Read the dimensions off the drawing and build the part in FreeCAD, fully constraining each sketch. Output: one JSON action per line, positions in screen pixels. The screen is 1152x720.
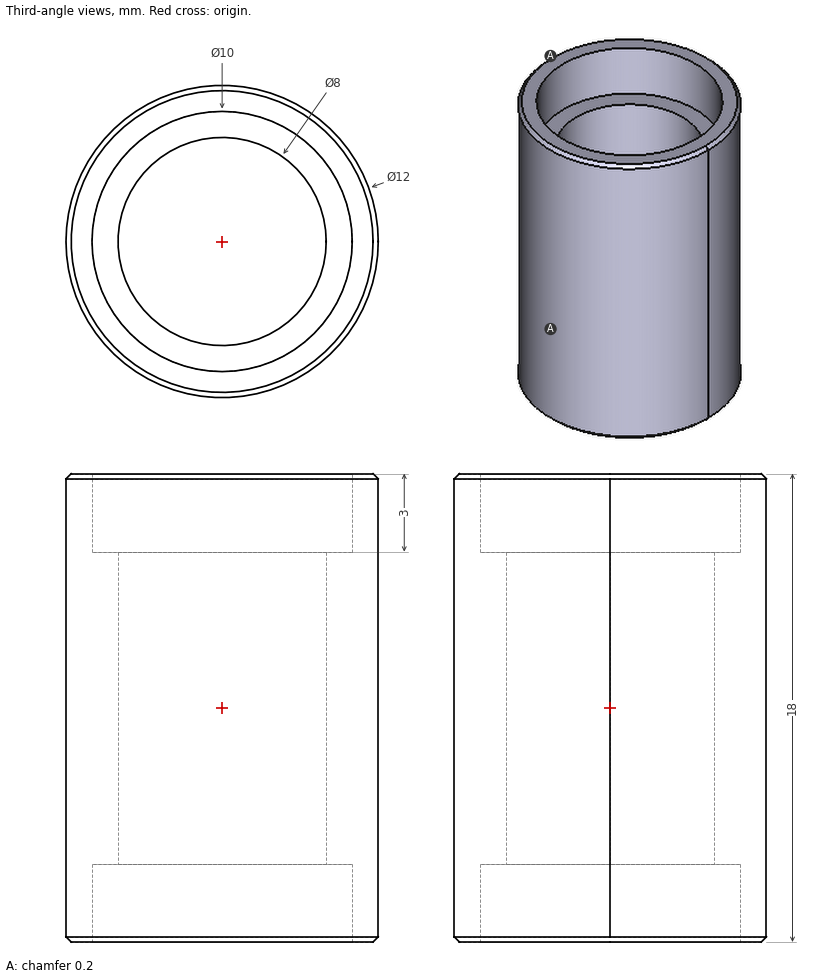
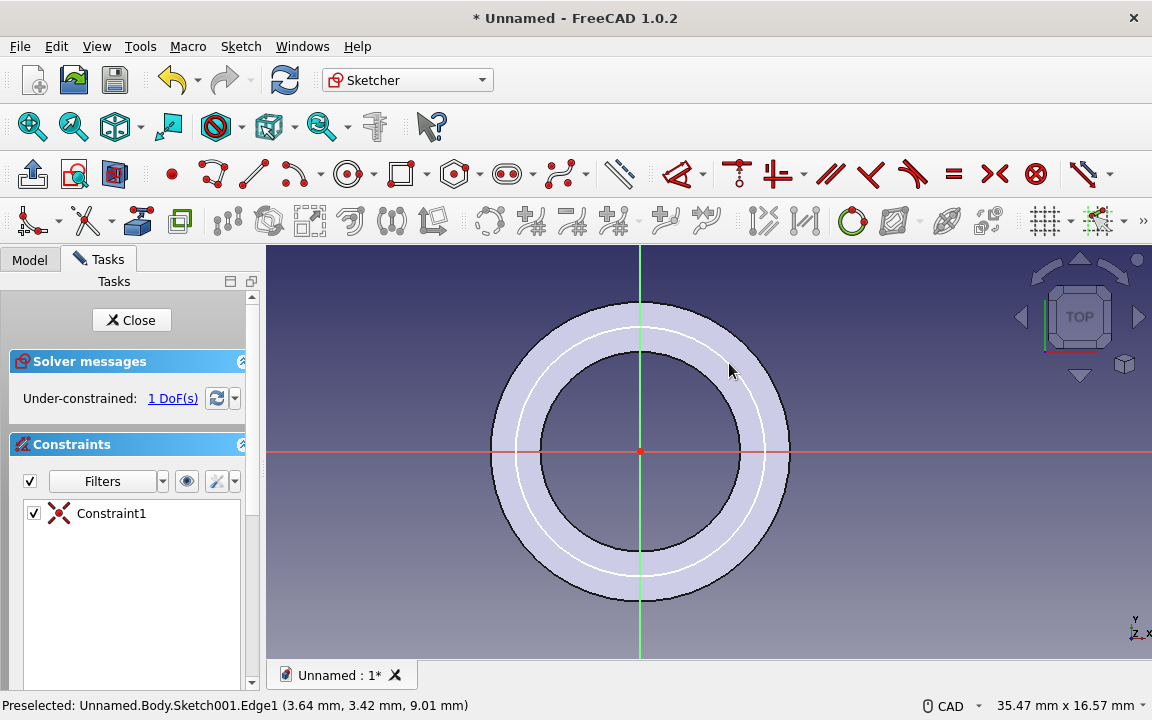
{"action": "left_click", "coordinate": [676, 174]}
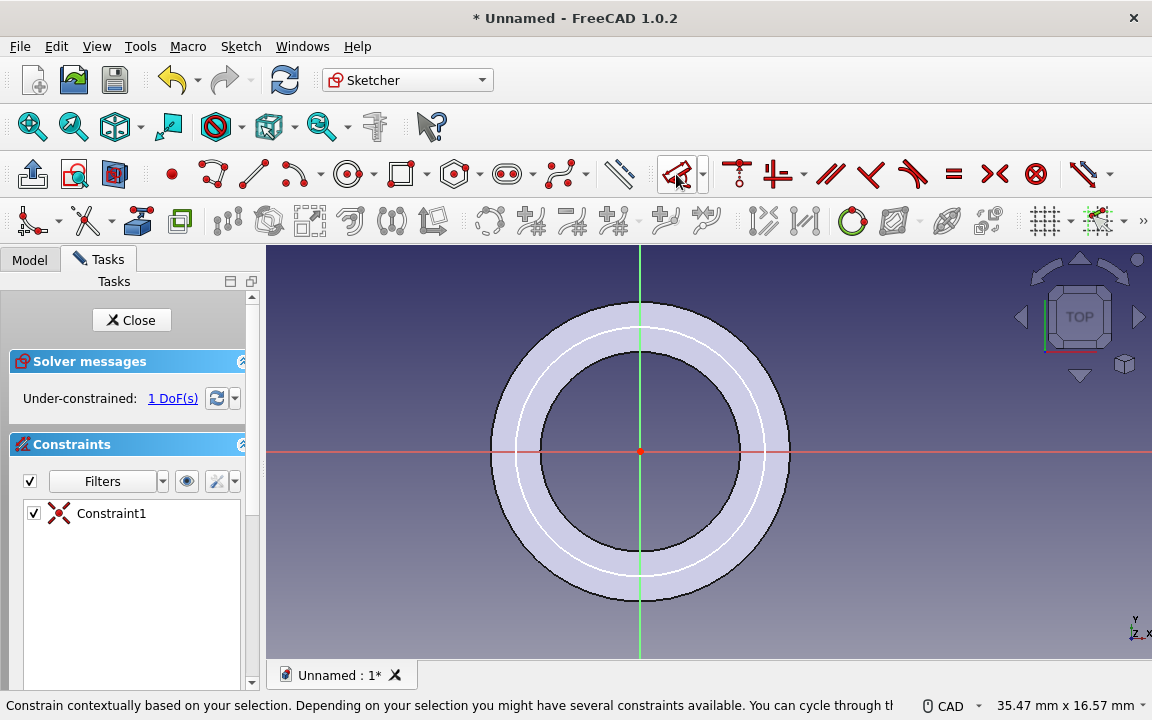
{"action": "left_click", "coordinate": [728, 363]}
{"action": "left_click", "coordinate": [750, 340]}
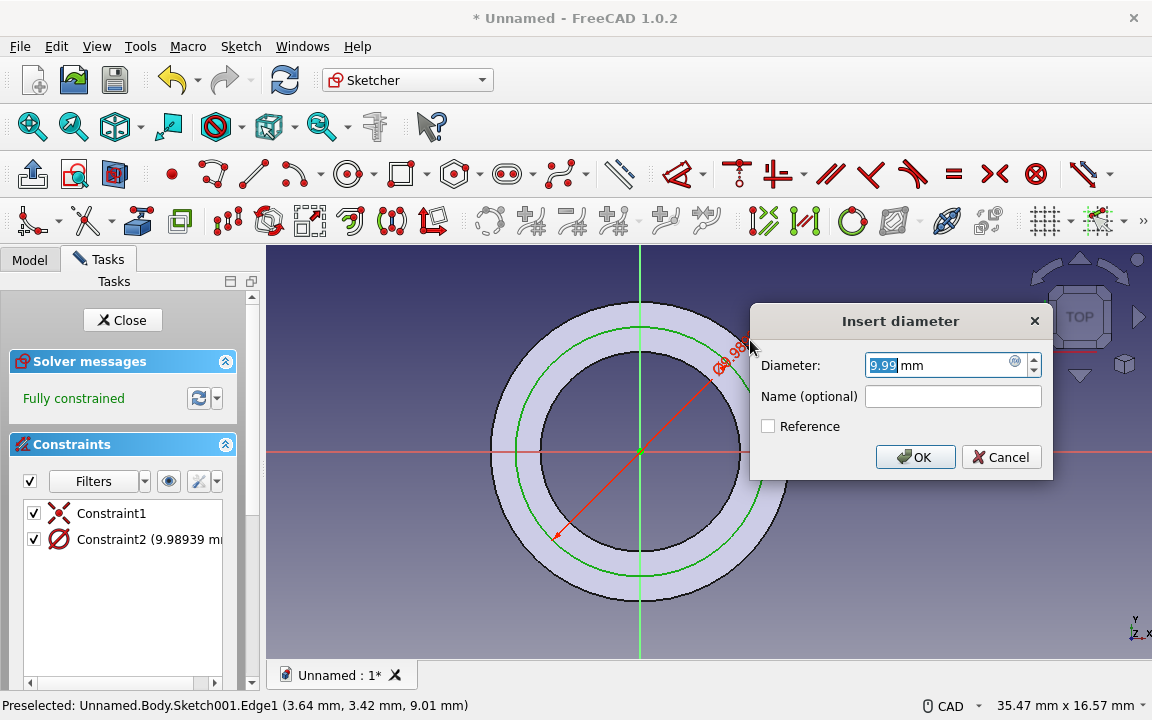
{"action": "type", "text": "10"}
{"action": "key", "text": "Return"}
{"action": "key", "text": "Escape"}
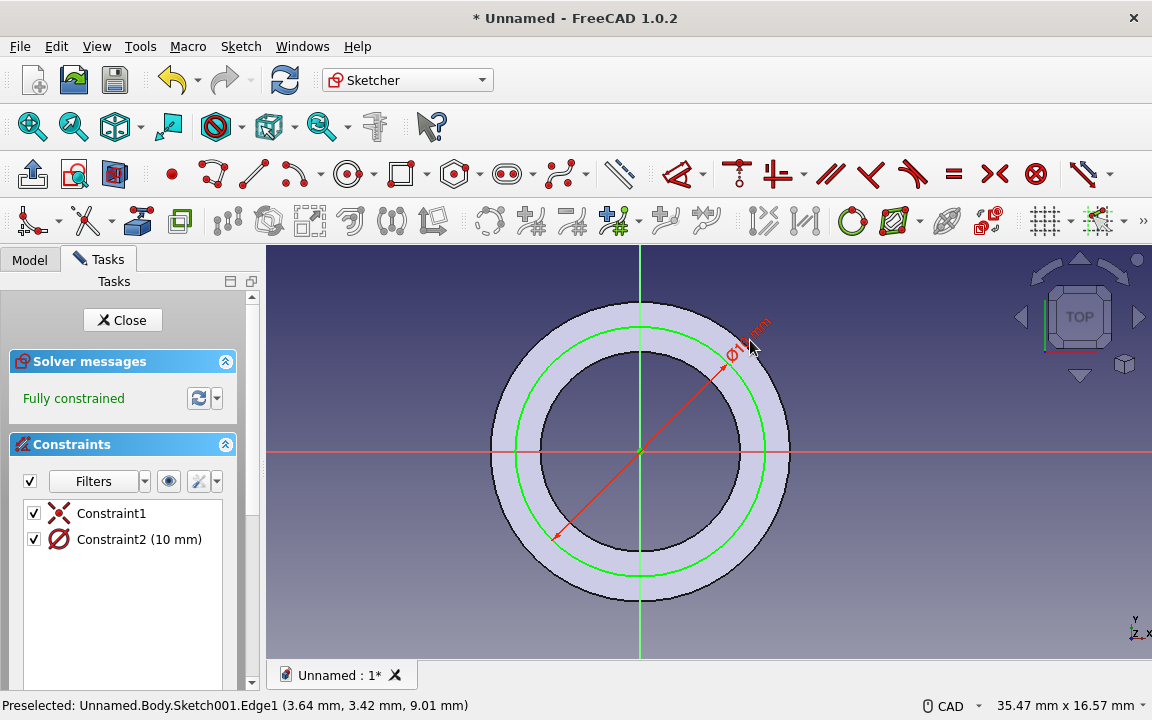
{"action": "left_click", "coordinate": [123, 320]}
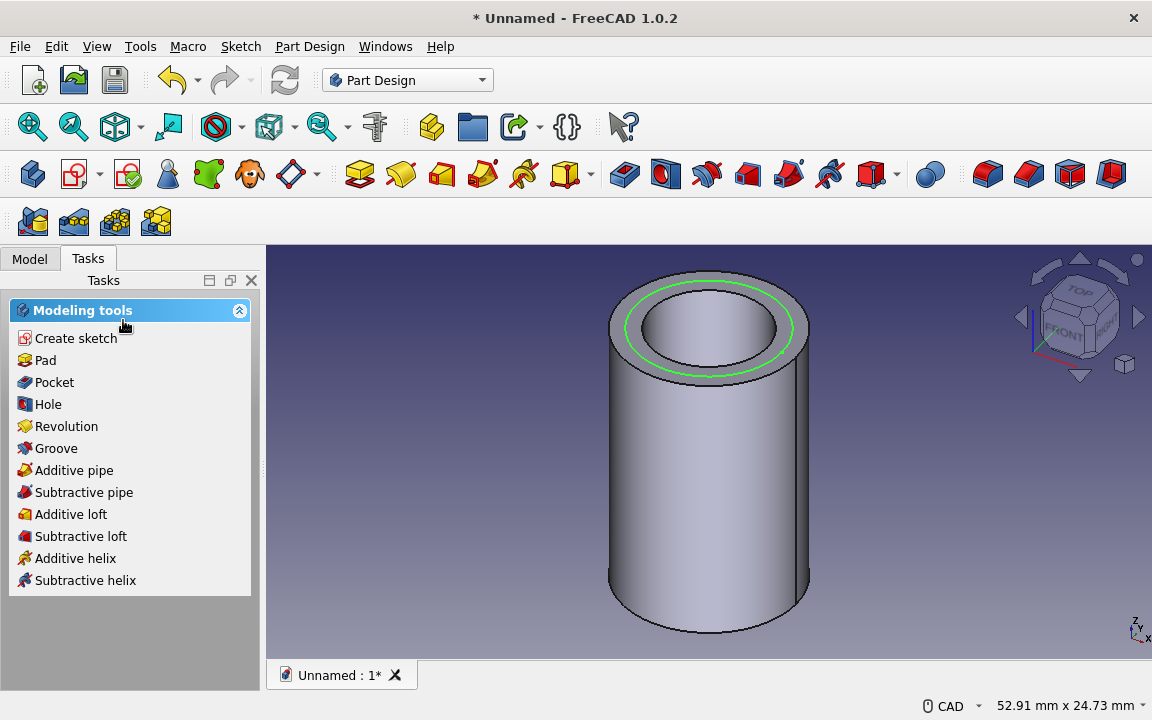
{"action": "left_click", "coordinate": [625, 174]}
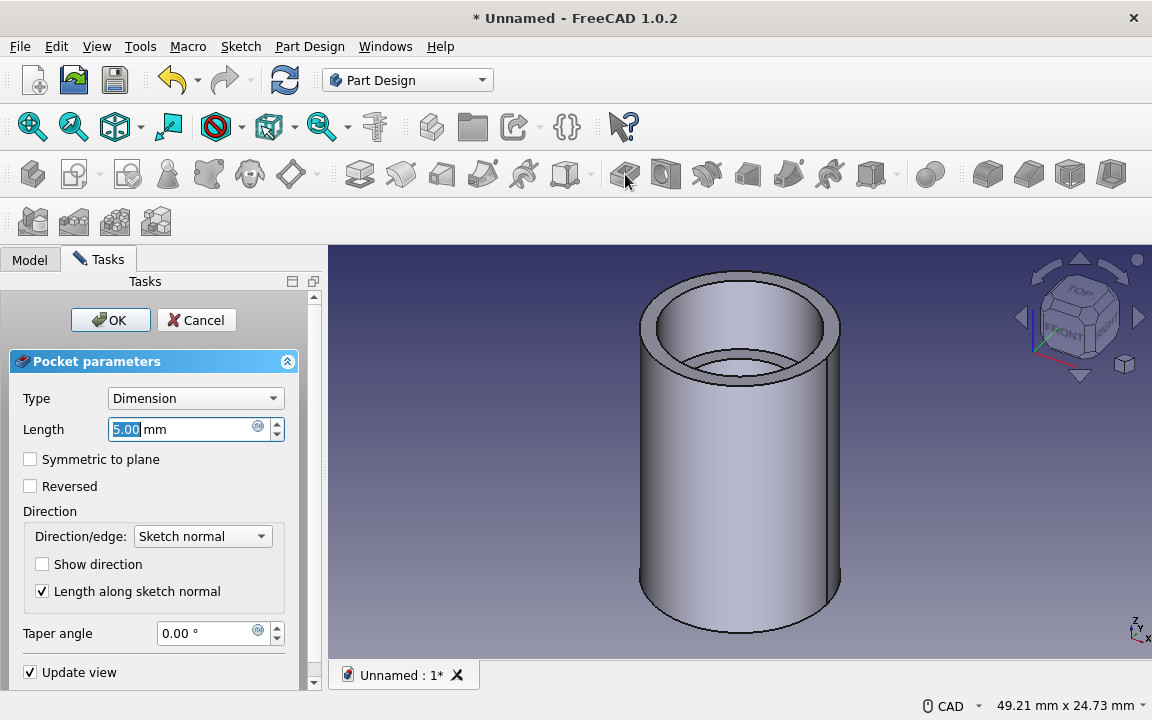
{"action": "type", "text": "3"}
{"action": "key", "text": "Tab"}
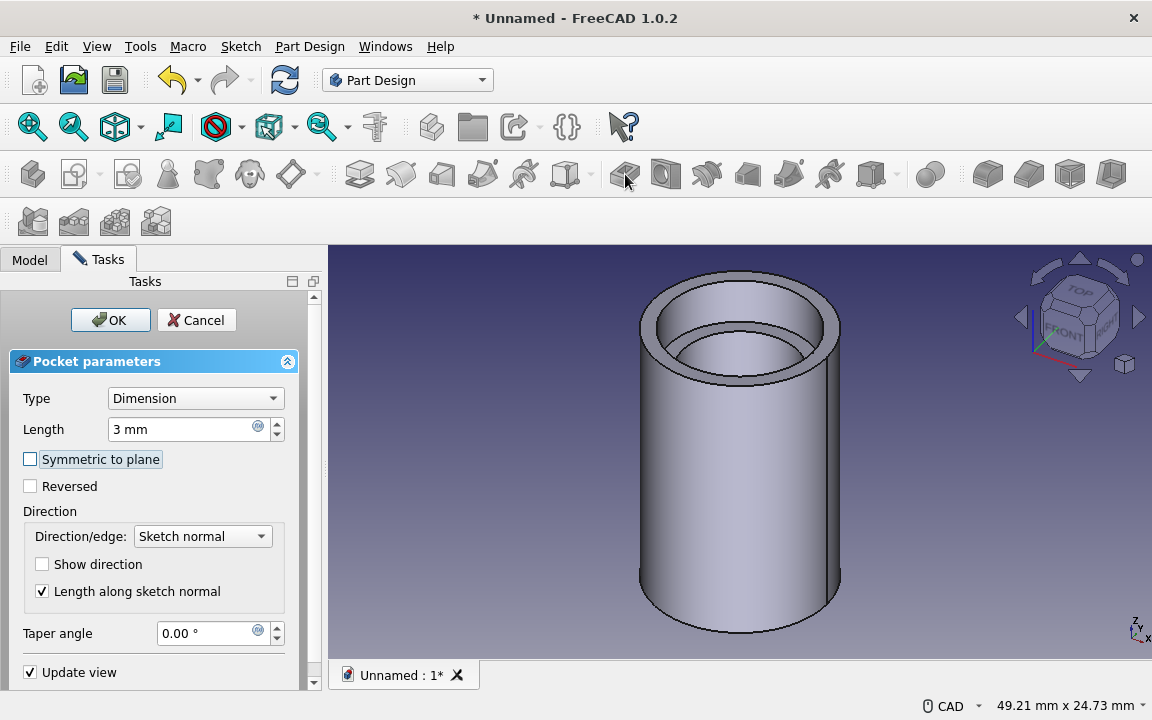
{"action": "left_click", "coordinate": [111, 320]}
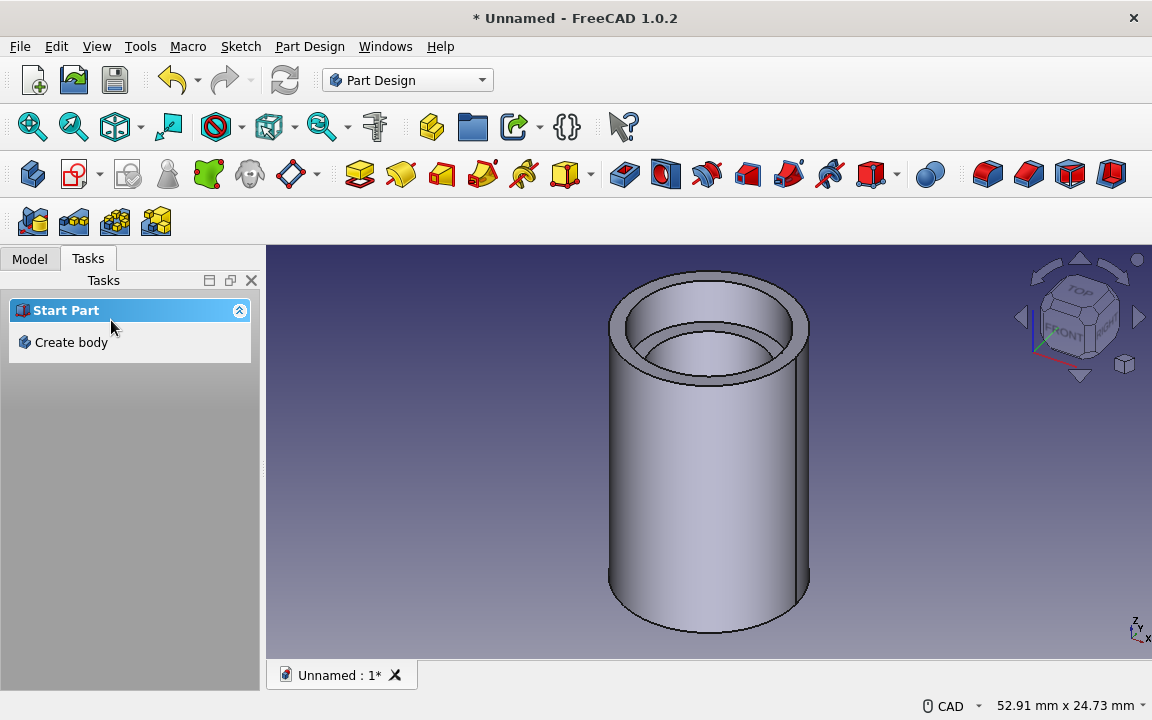
{"action": "left_click", "coordinate": [30, 258]}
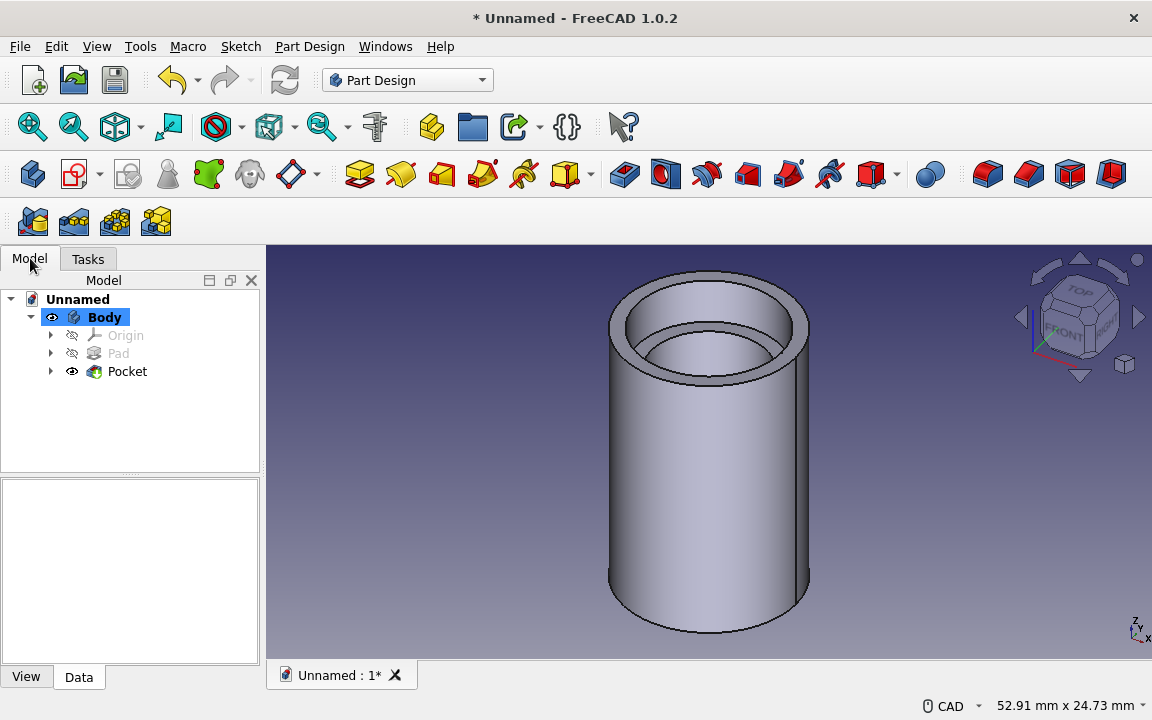
{"action": "left_click", "coordinate": [117, 371]}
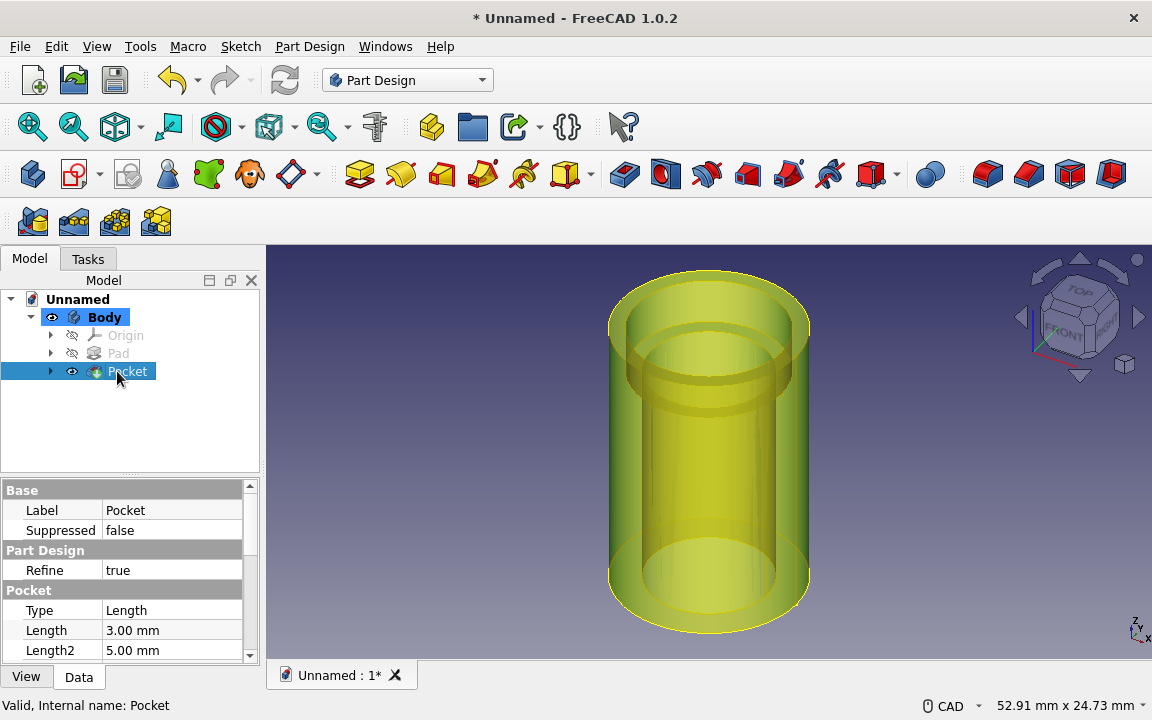
{"action": "left_click", "coordinate": [33, 222]}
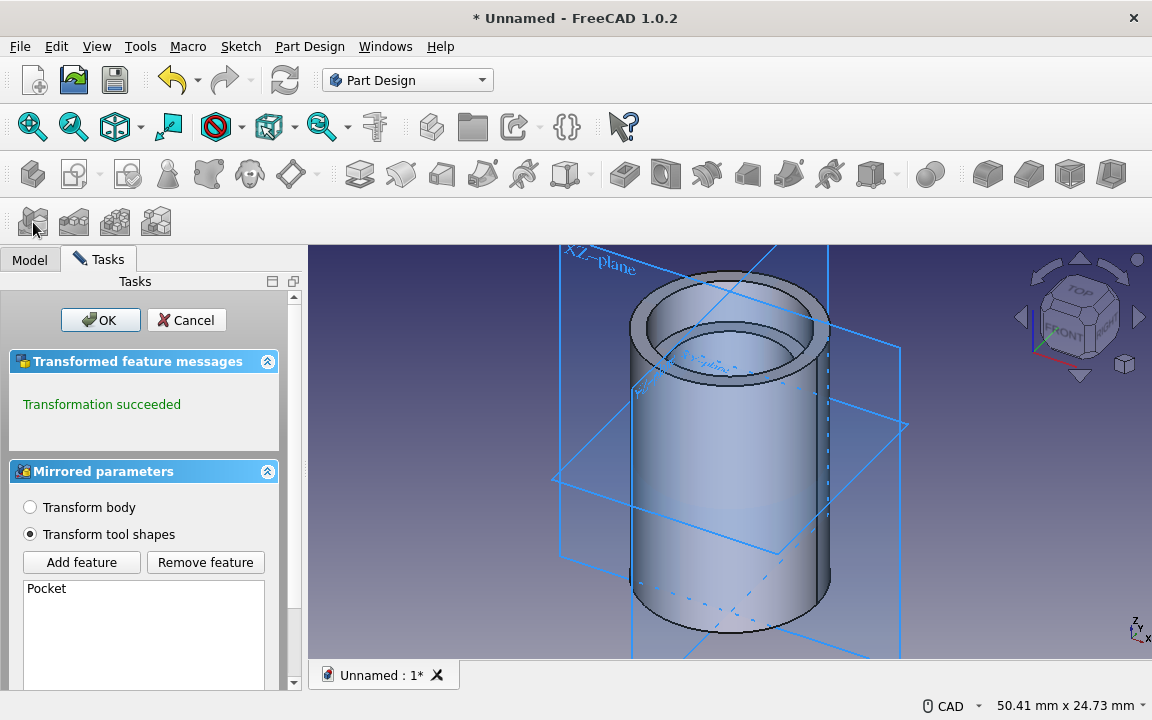
{"action": "scroll", "coordinate": [294, 490], "scroll_direction": "down", "scroll_amount": 2}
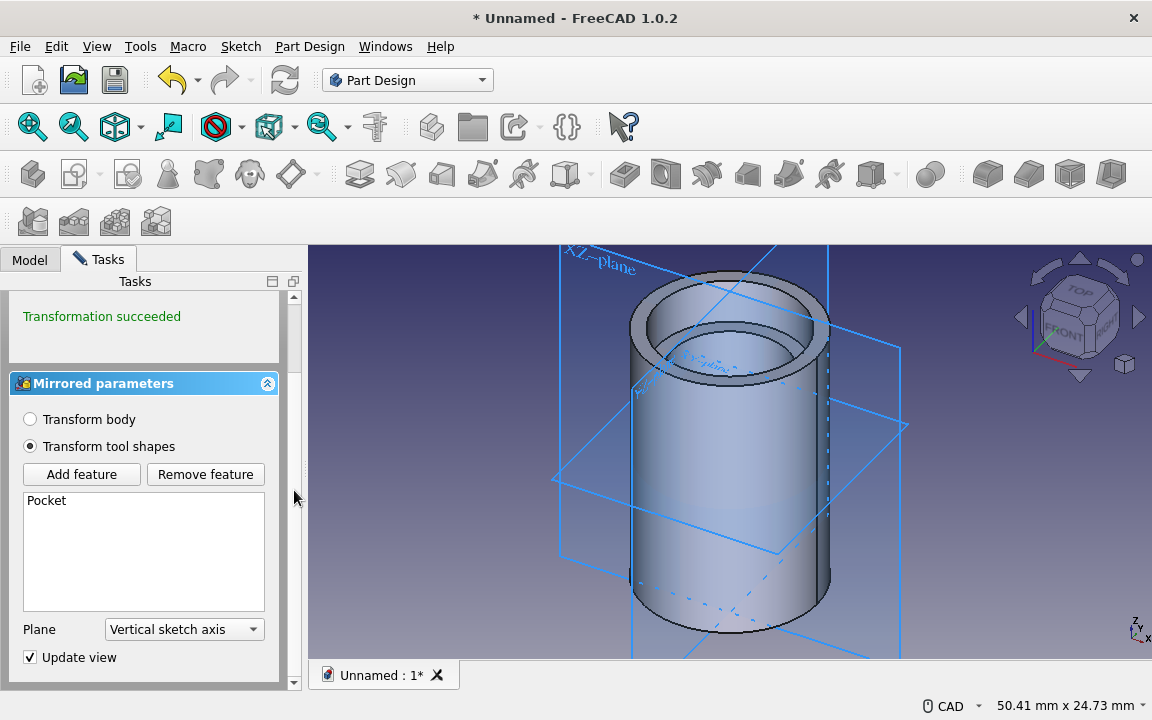
{"action": "left_click", "coordinate": [185, 630]}